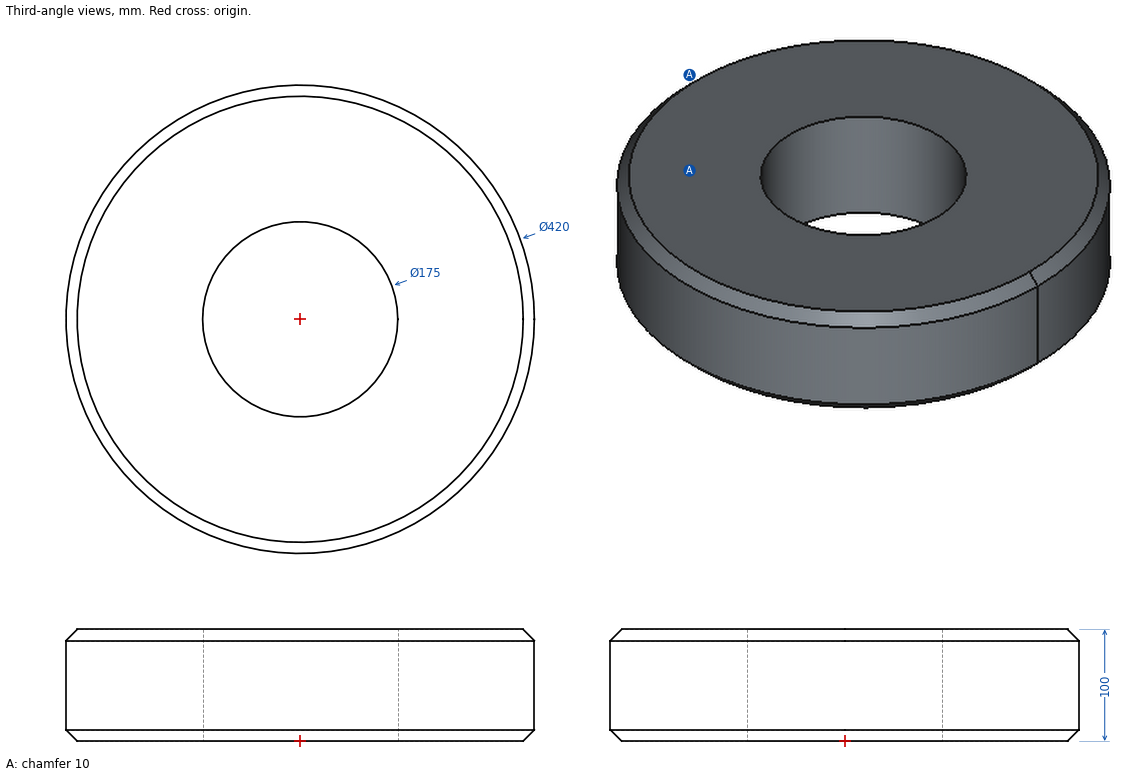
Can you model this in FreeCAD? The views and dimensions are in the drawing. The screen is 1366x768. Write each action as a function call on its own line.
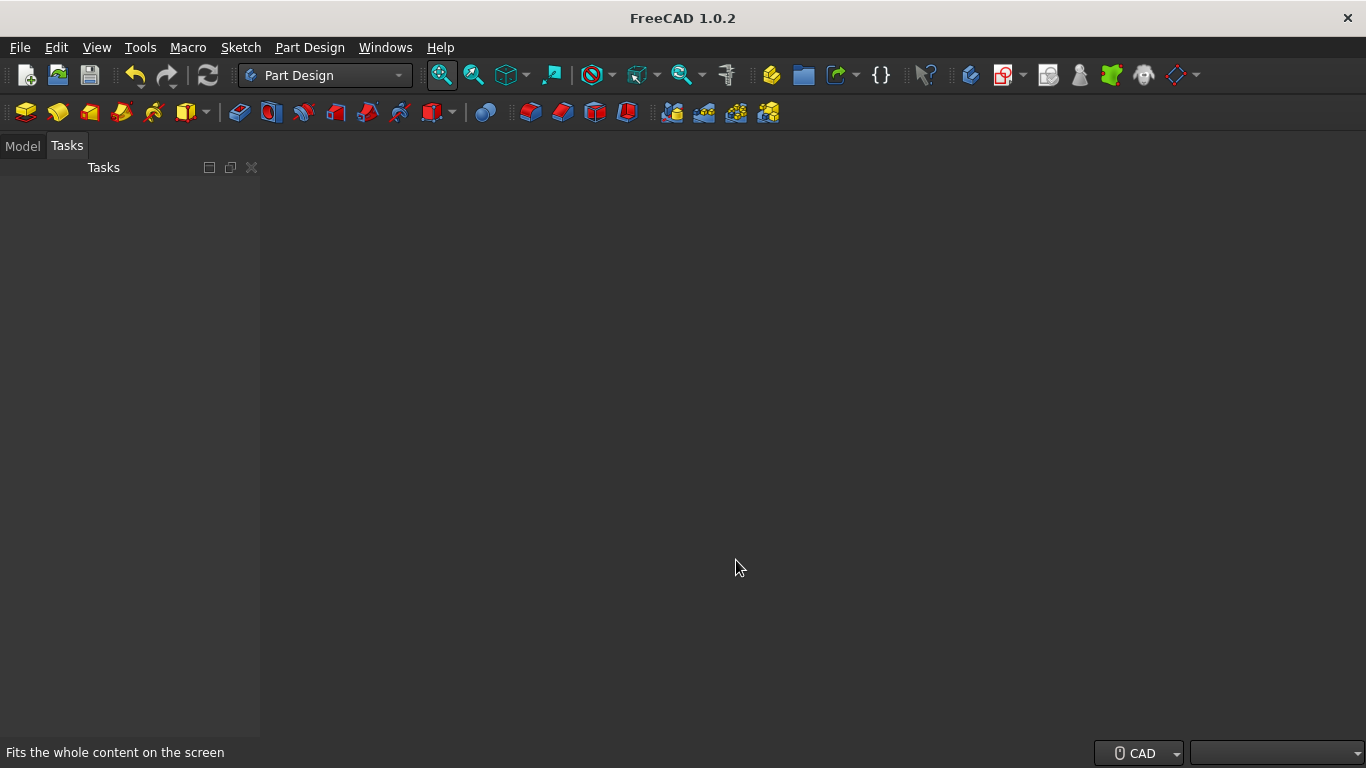
key(ctrl+n)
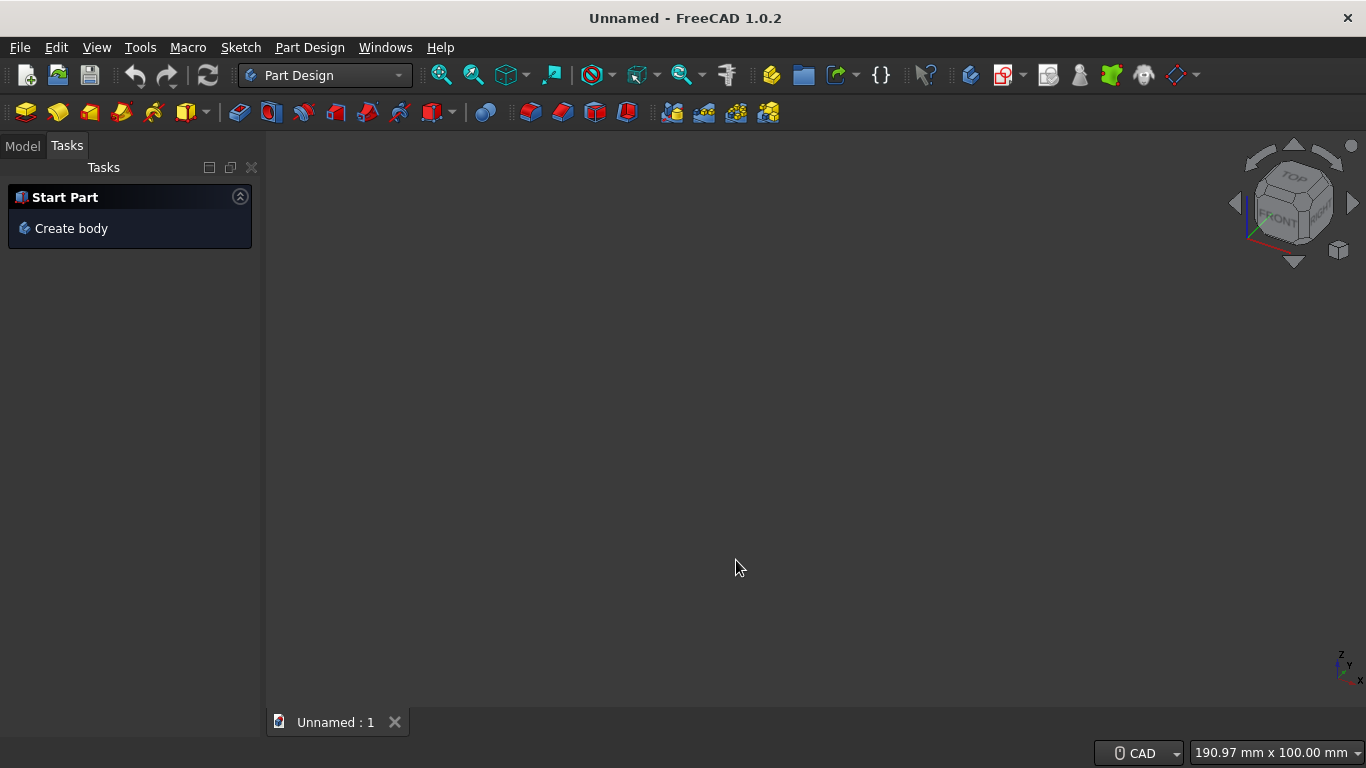
click(1004, 76)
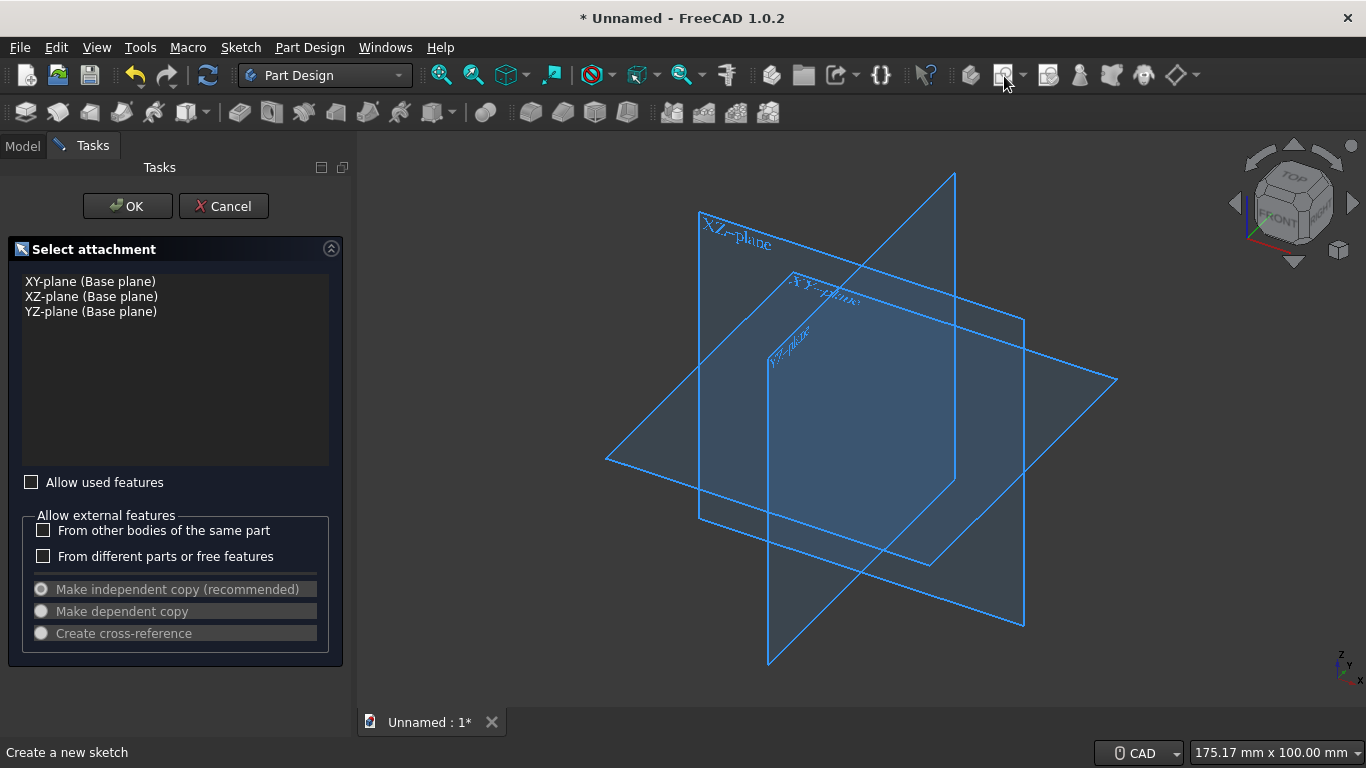
click(82, 282)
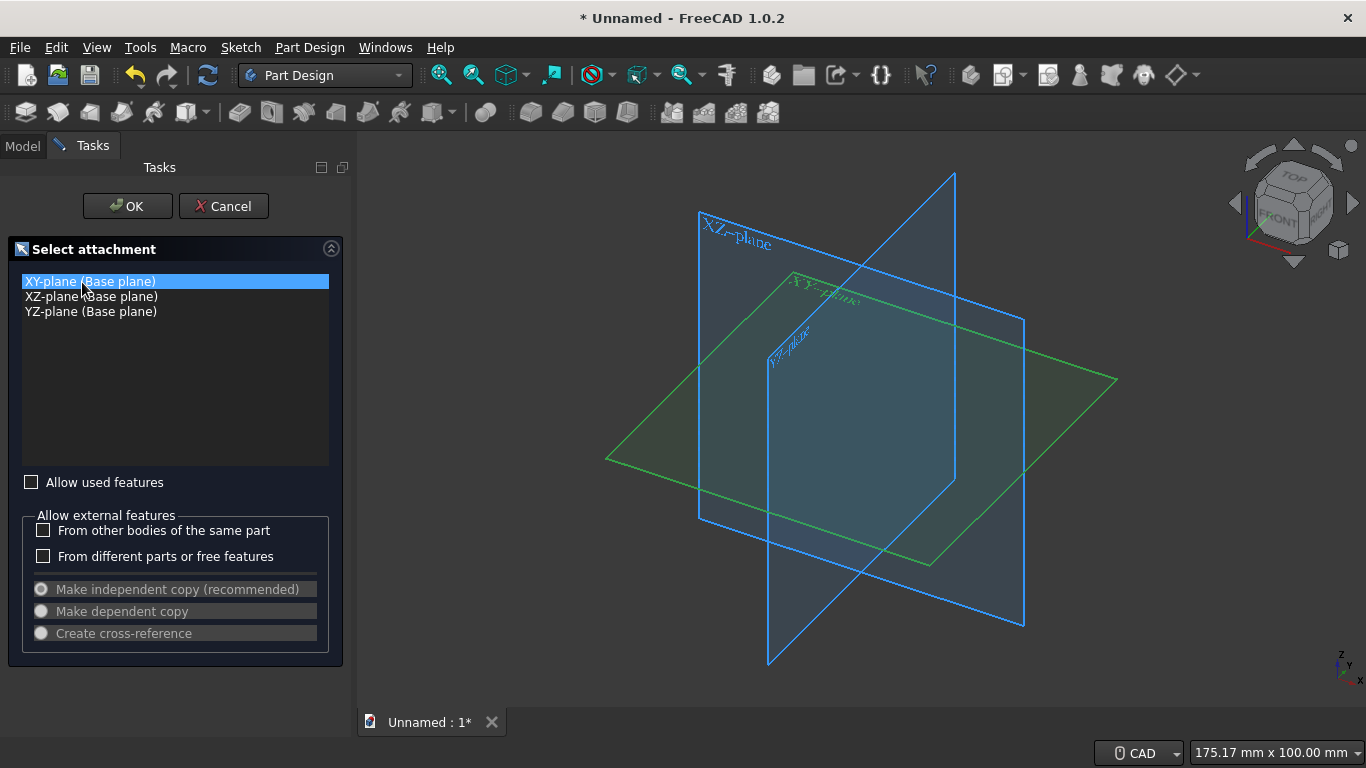
click(128, 206)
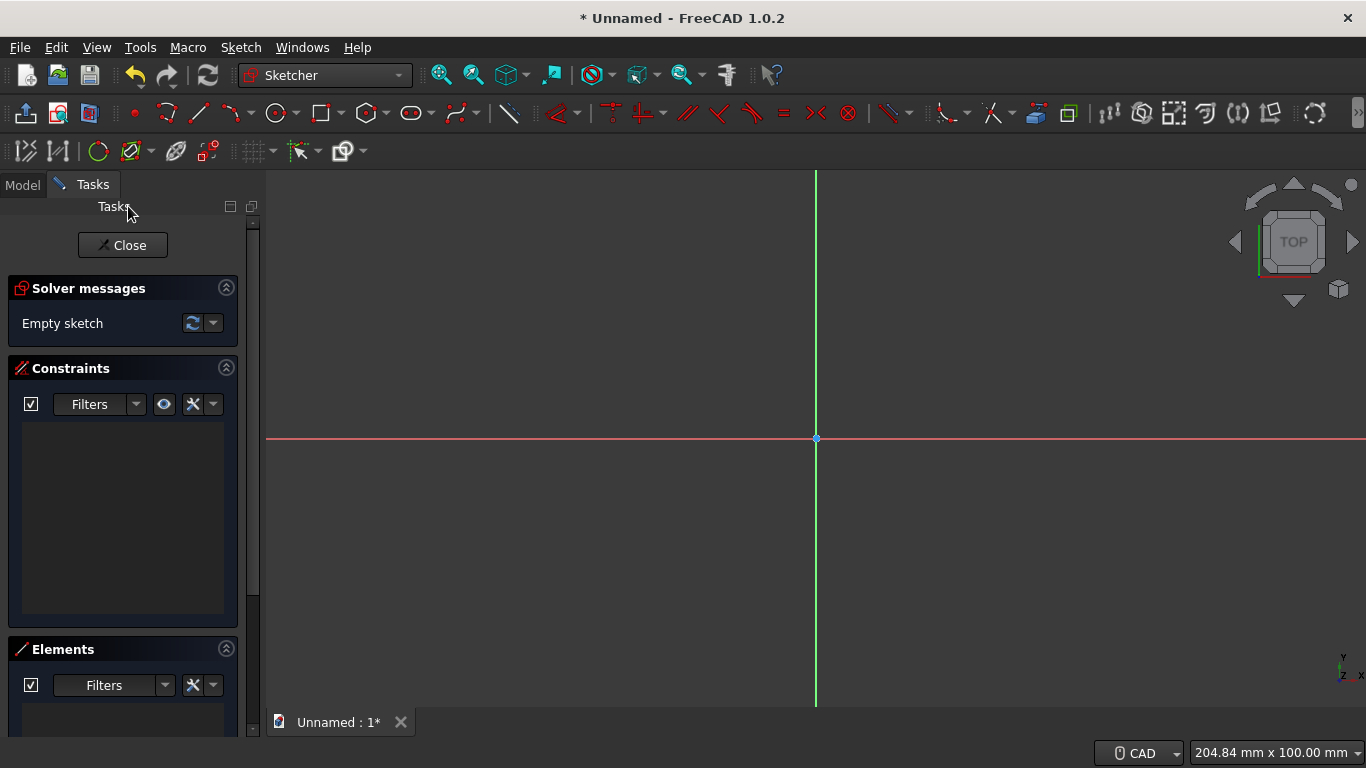
scroll(734, 438, down, 9)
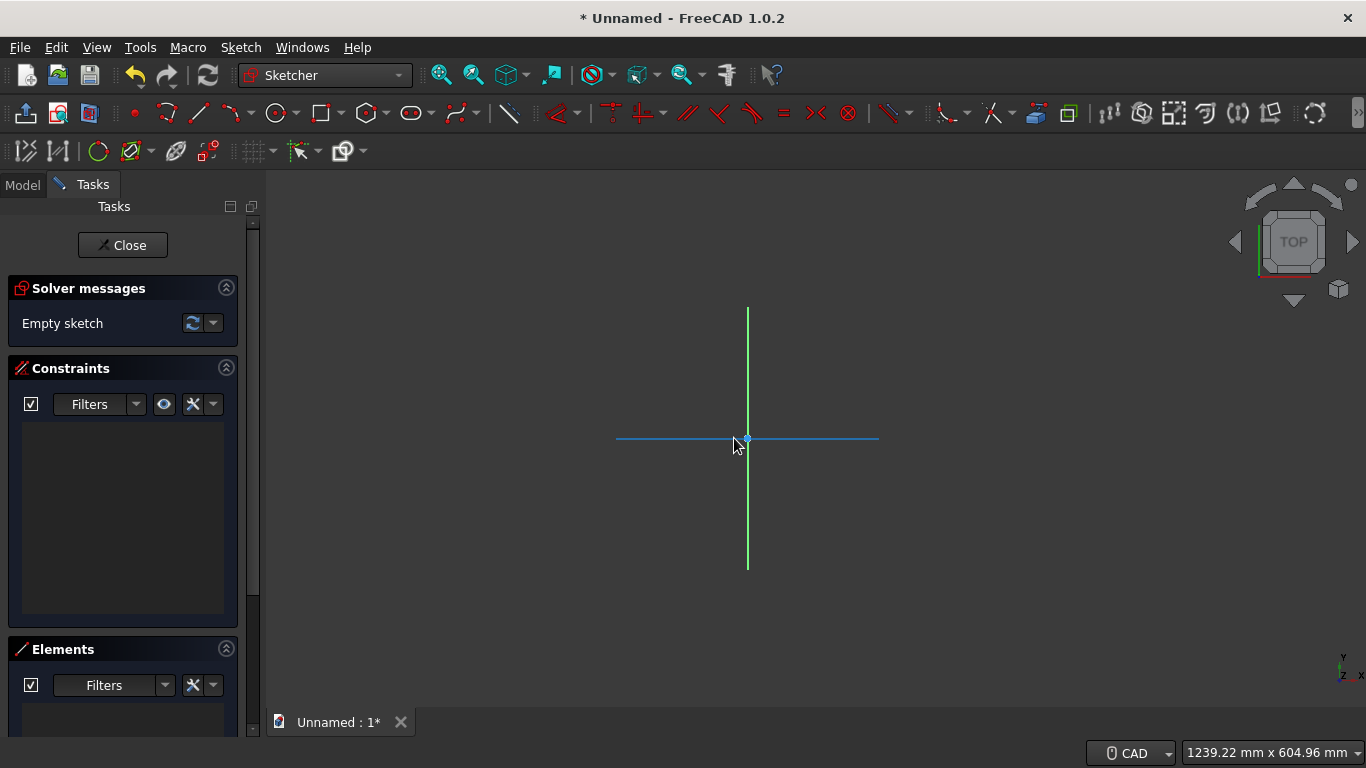
click(276, 114)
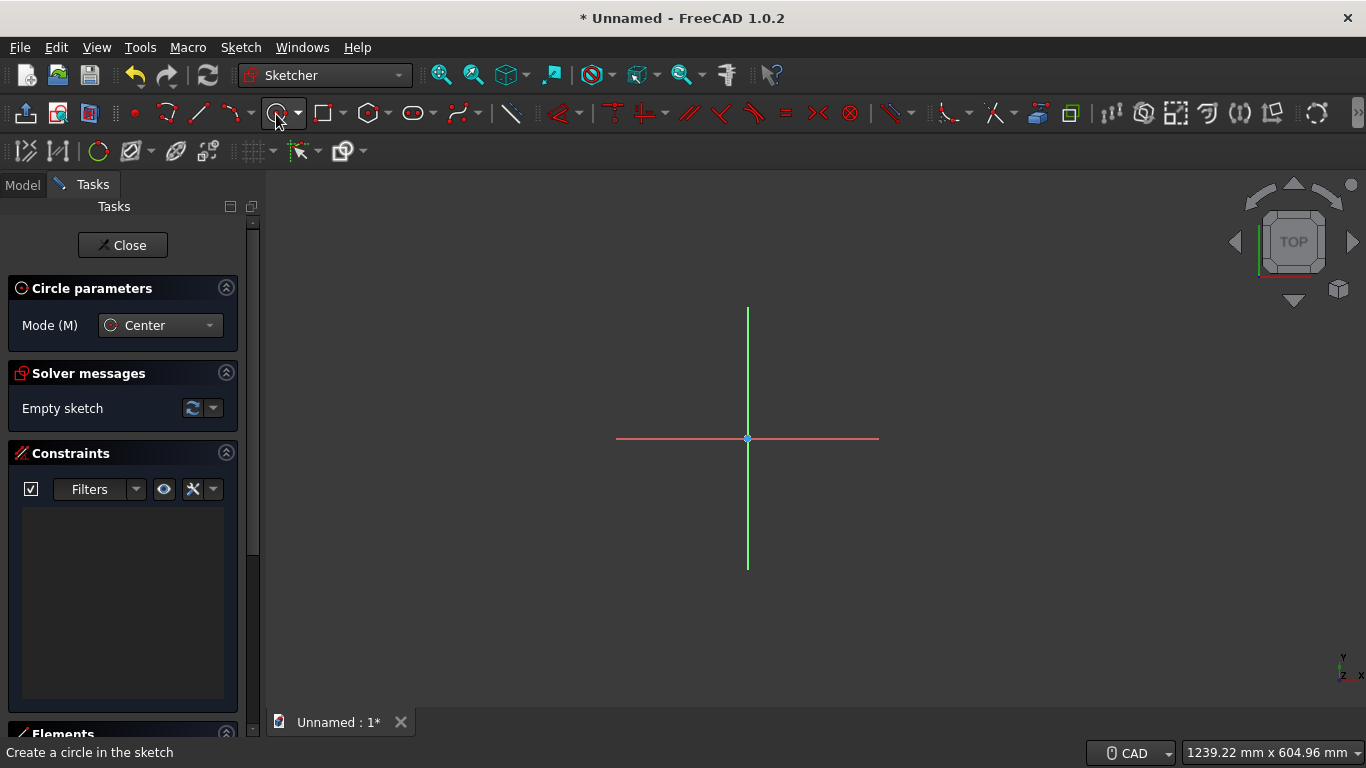
click(748, 438)
click(880, 307)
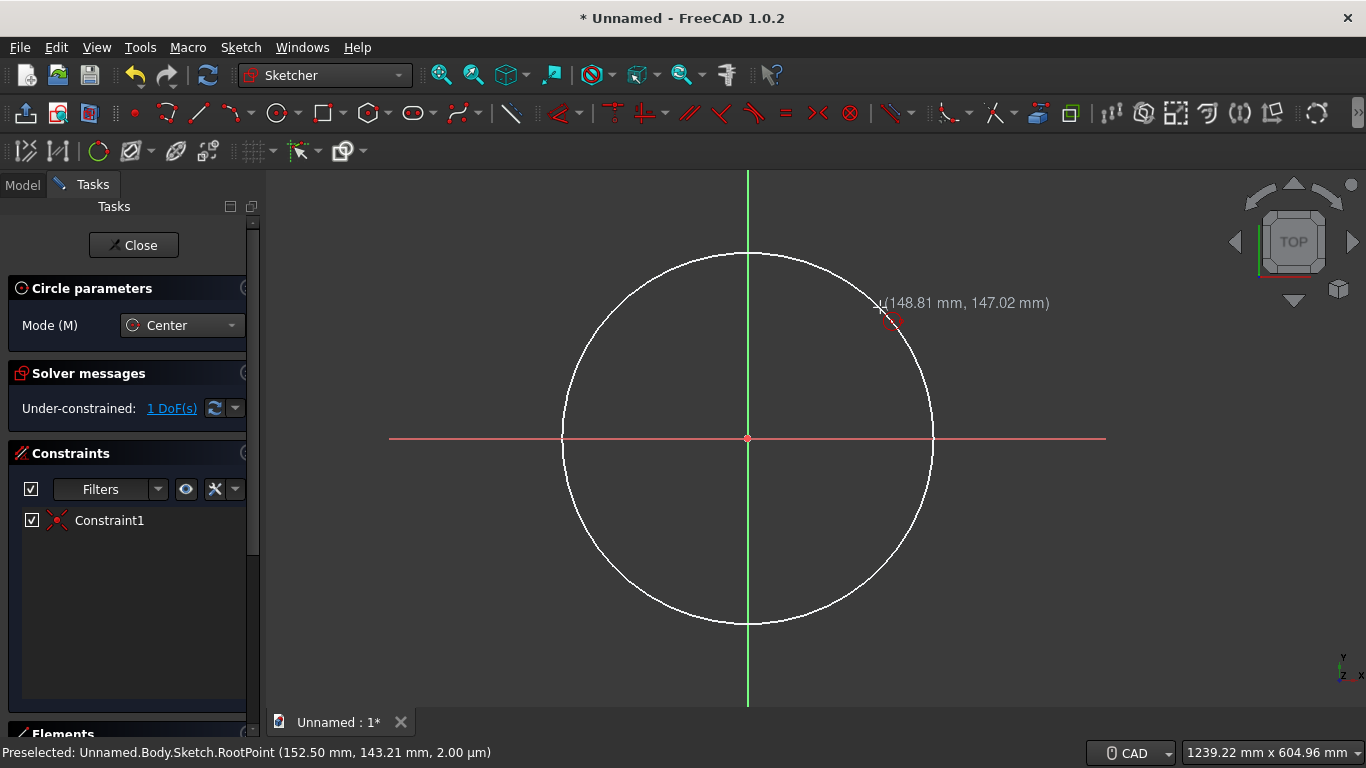
click(748, 438)
click(803, 384)
key(Escape)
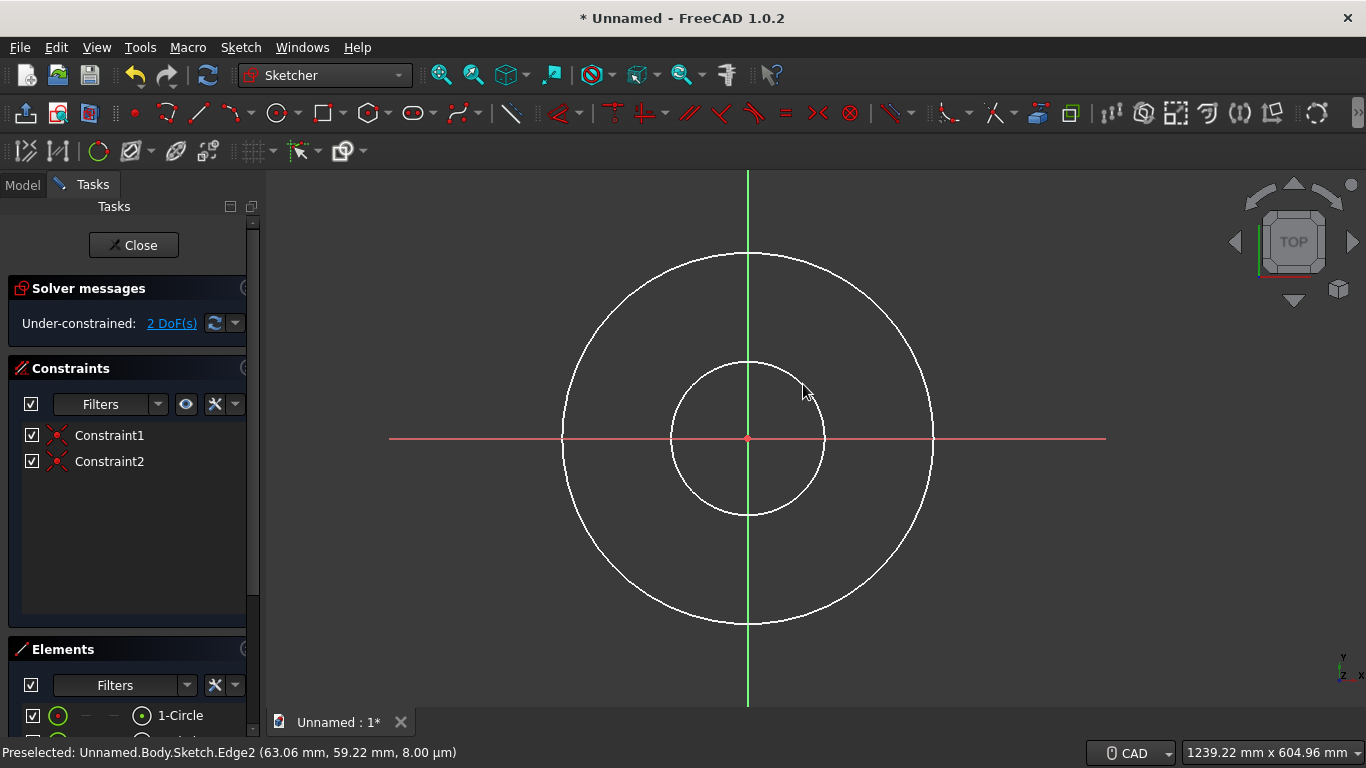
click(558, 114)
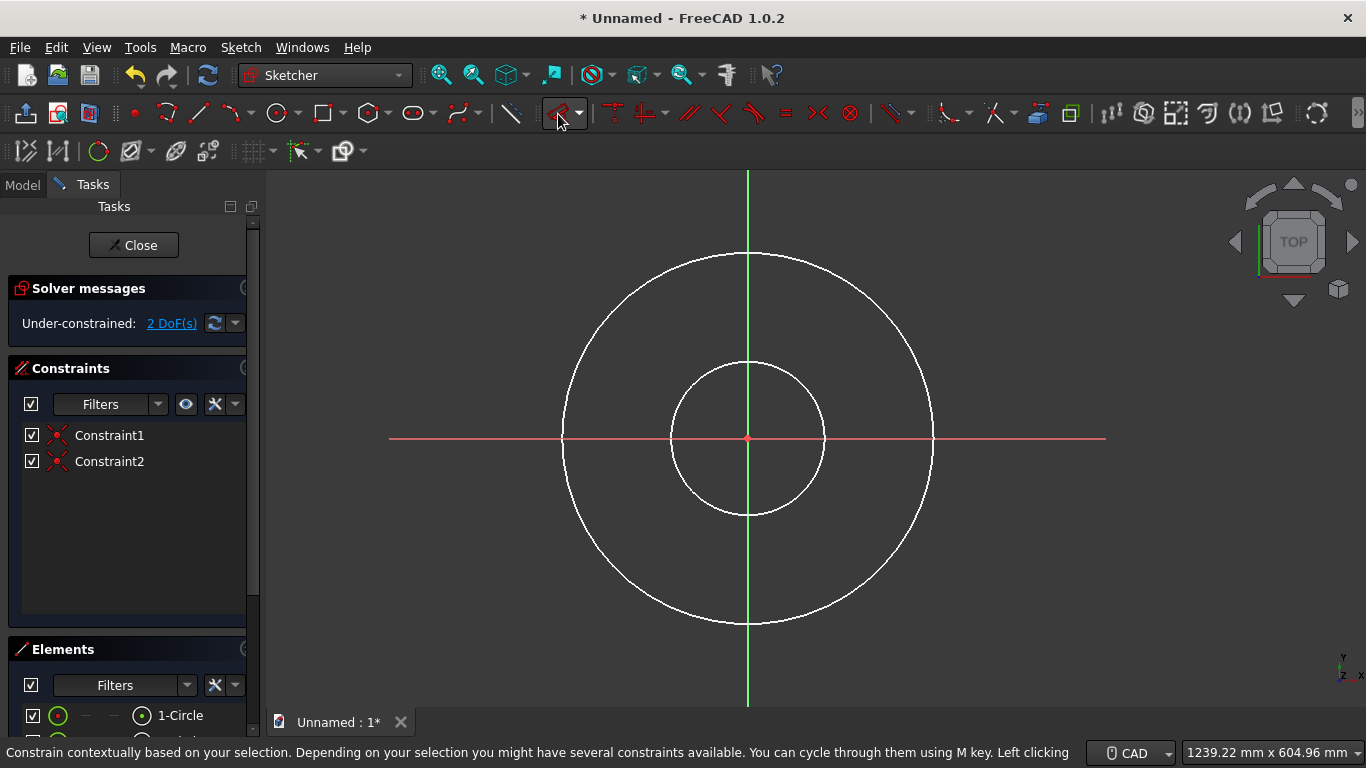
click(879, 307)
click(902, 284)